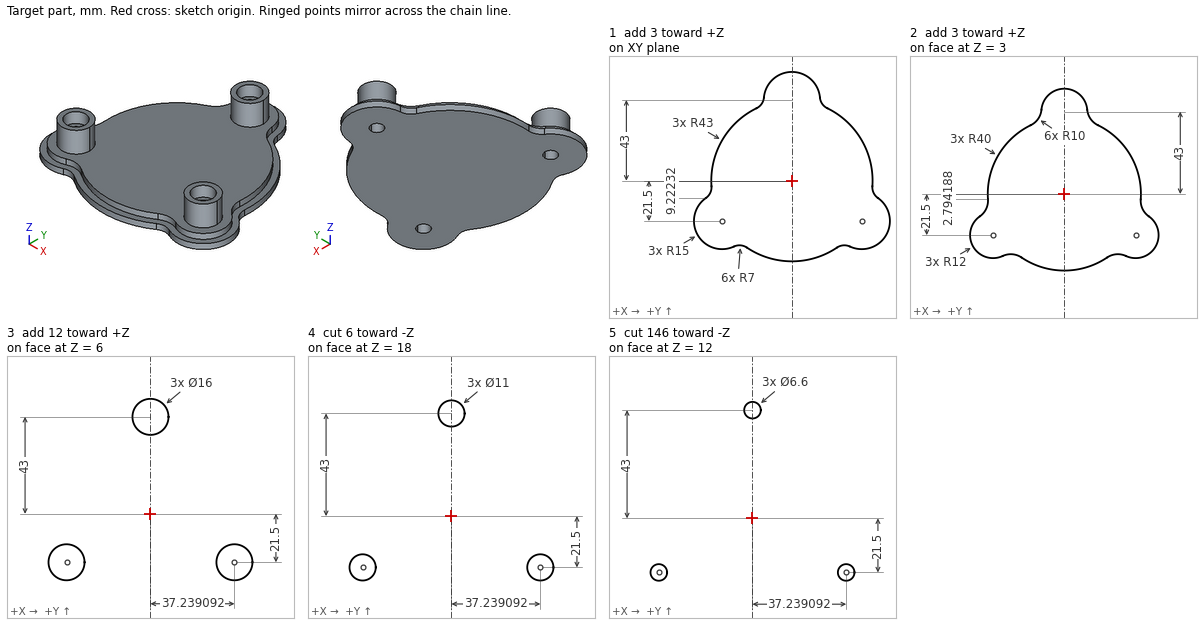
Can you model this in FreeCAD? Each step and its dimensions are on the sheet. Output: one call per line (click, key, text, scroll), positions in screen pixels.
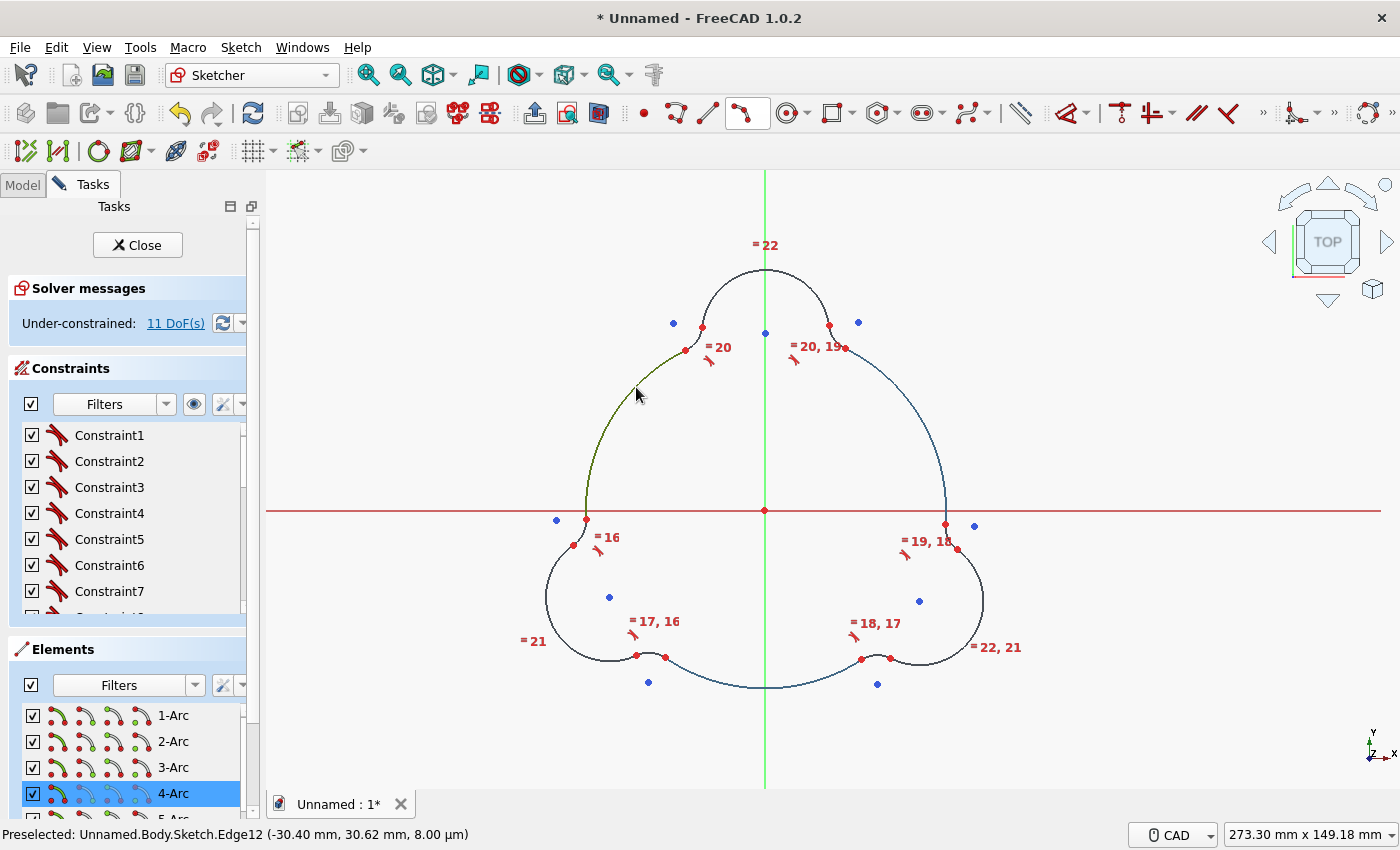
key(e)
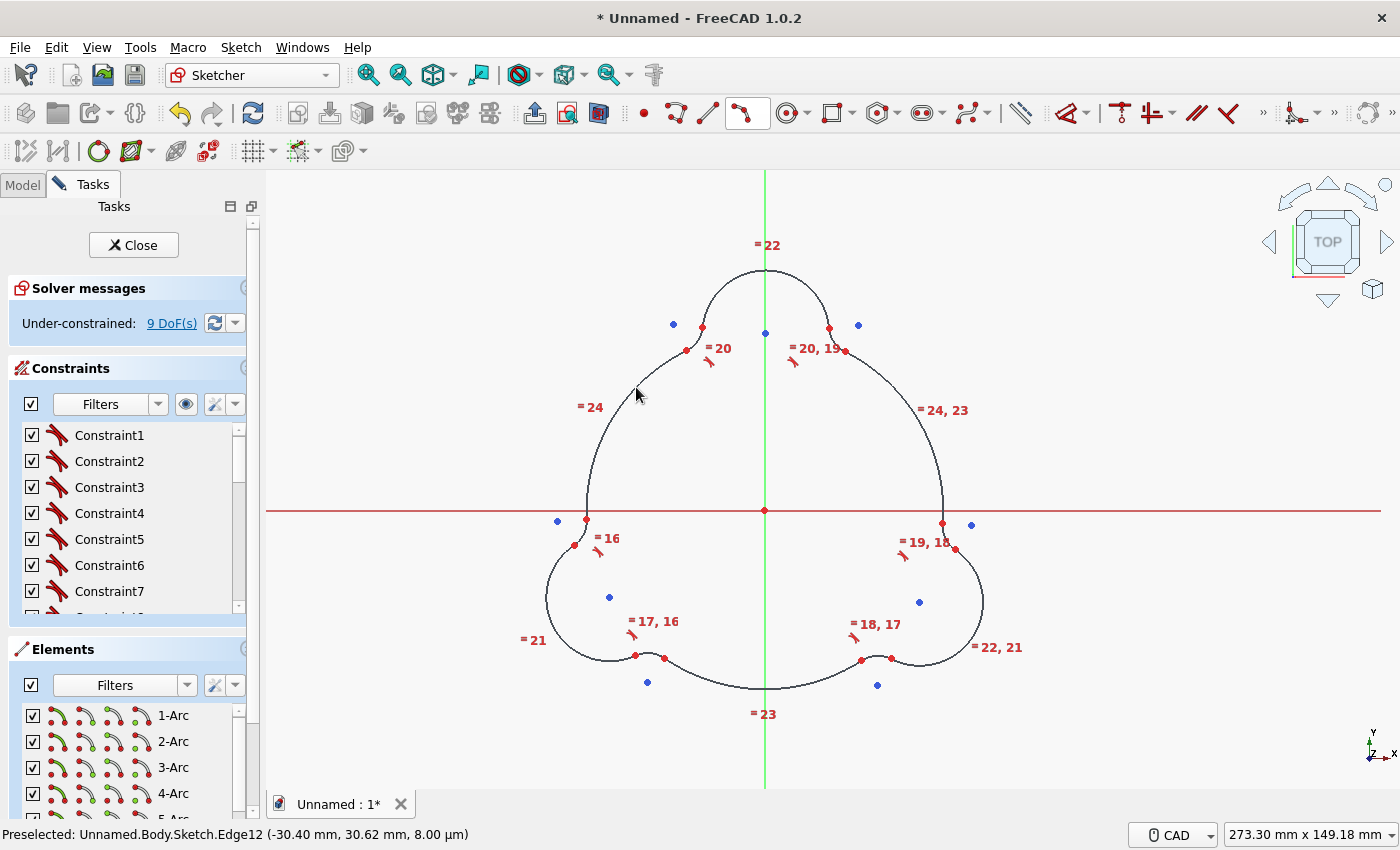
click(766, 334)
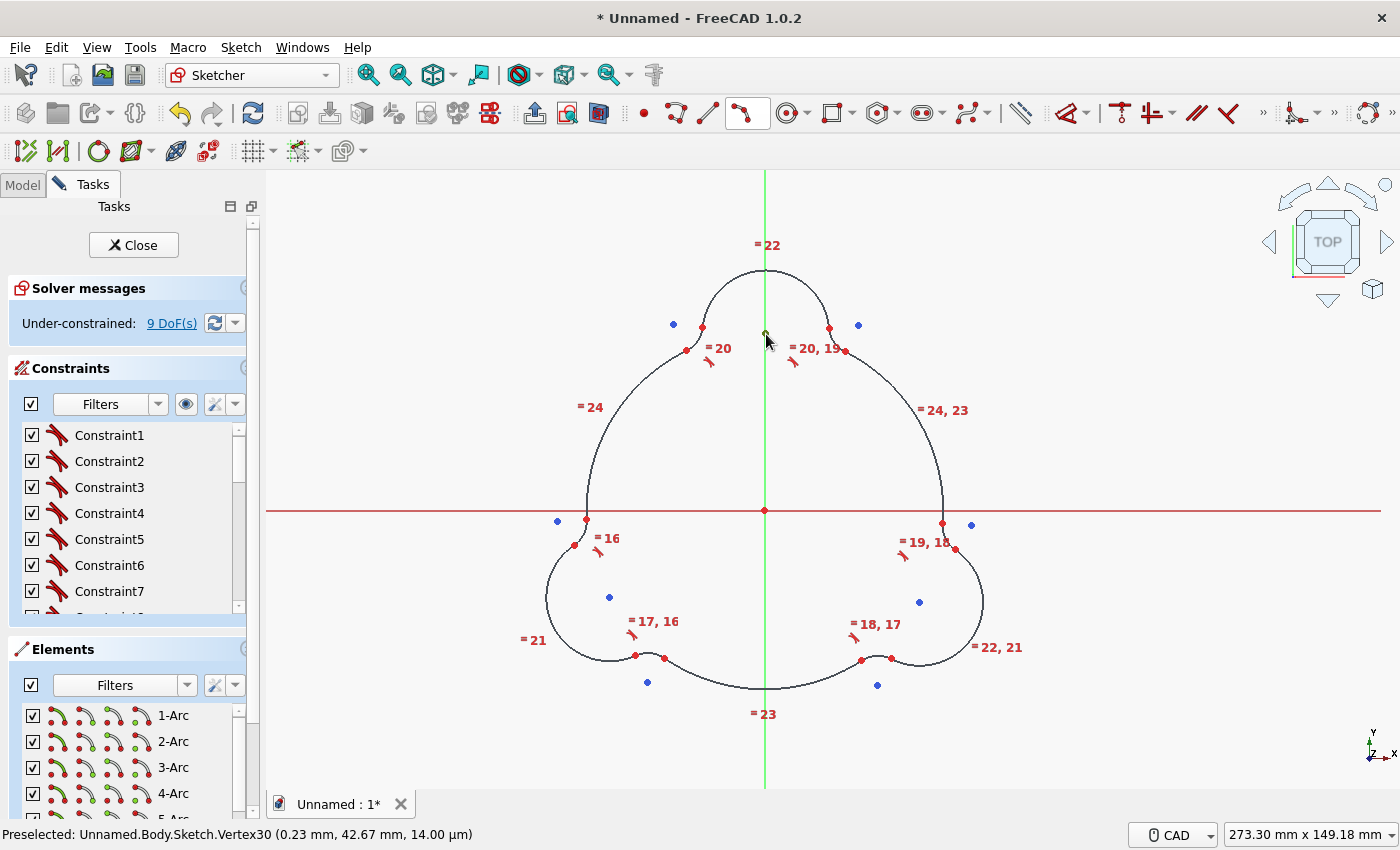
click(765, 721)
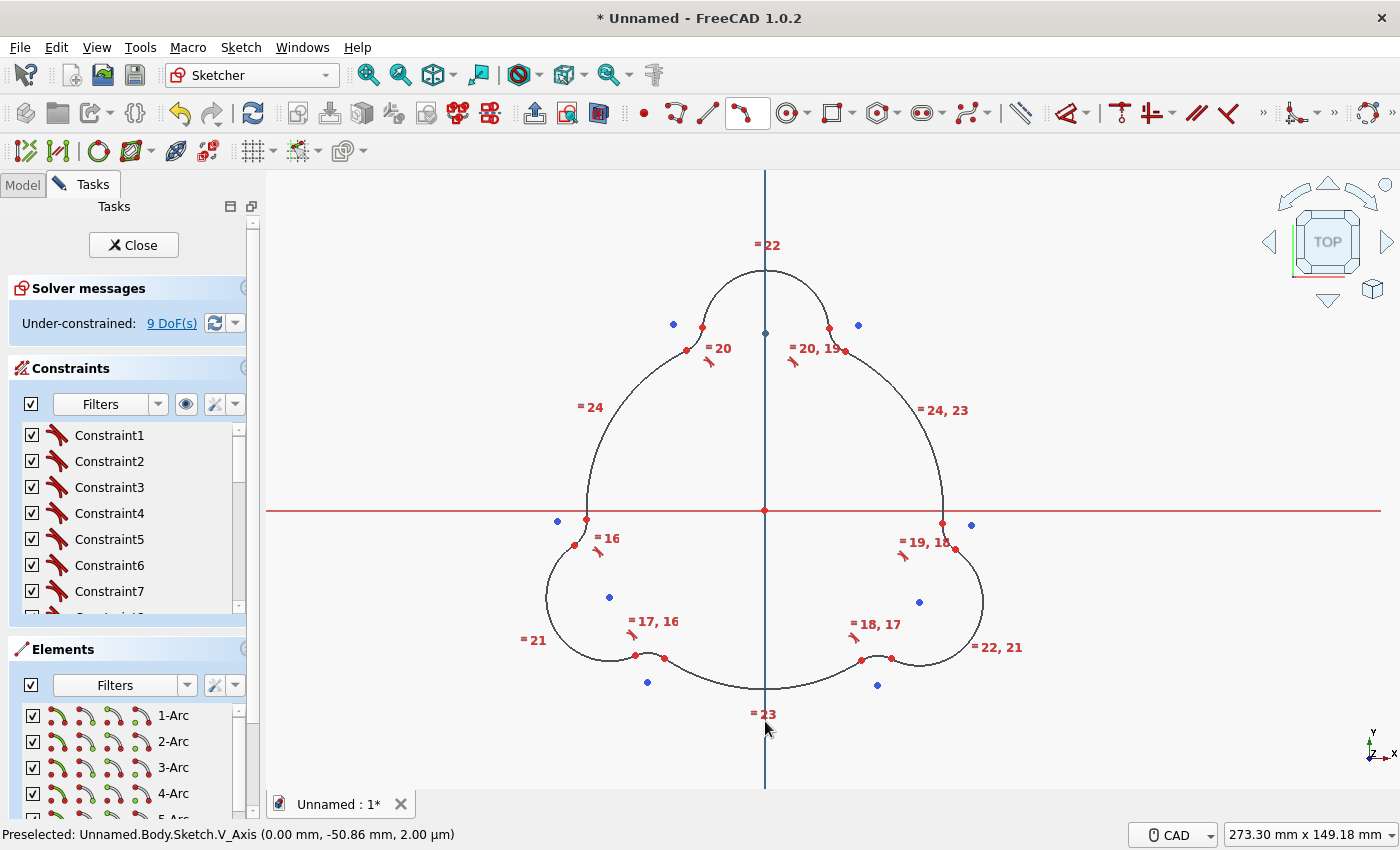
click(1120, 114)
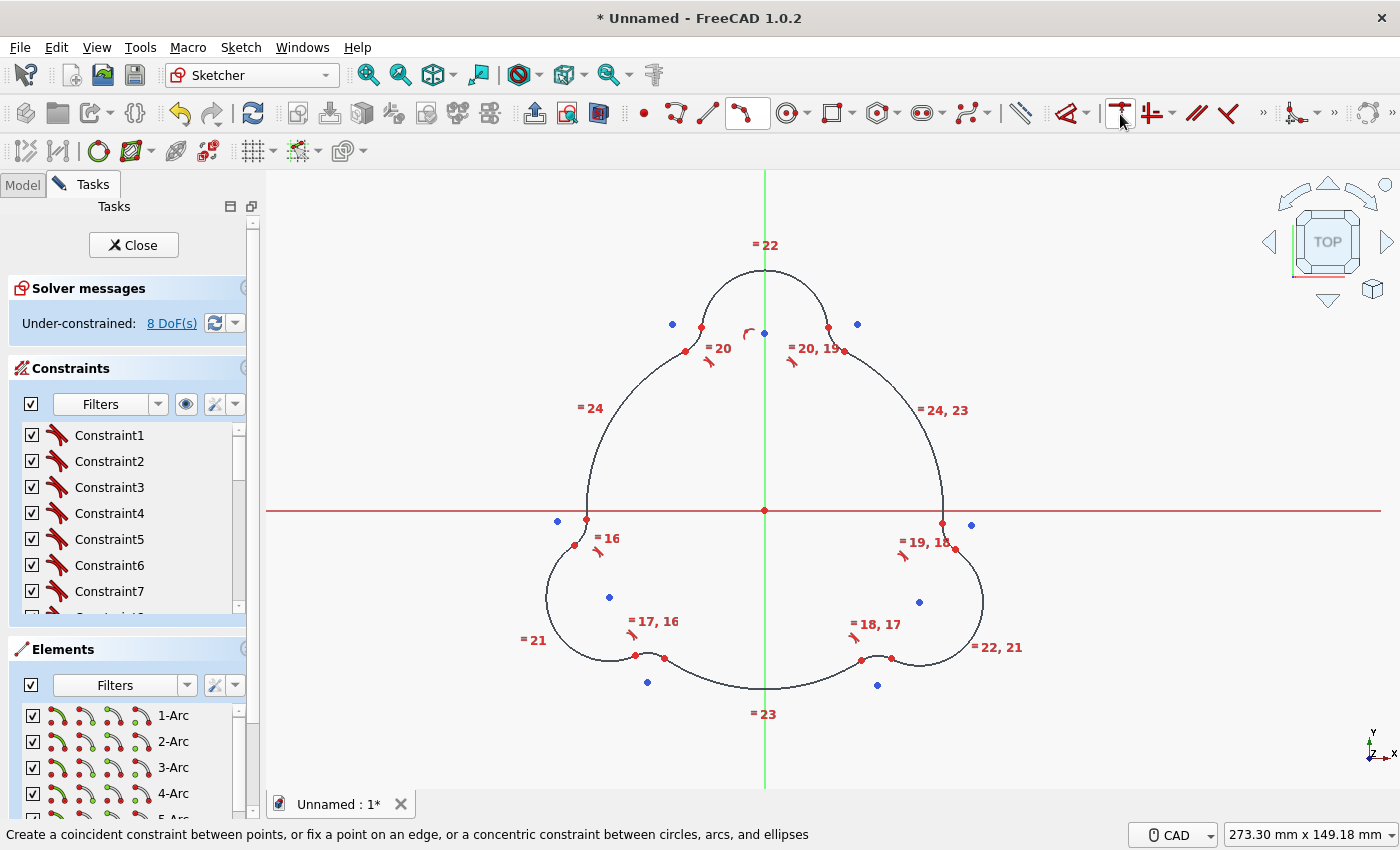
click(610, 598)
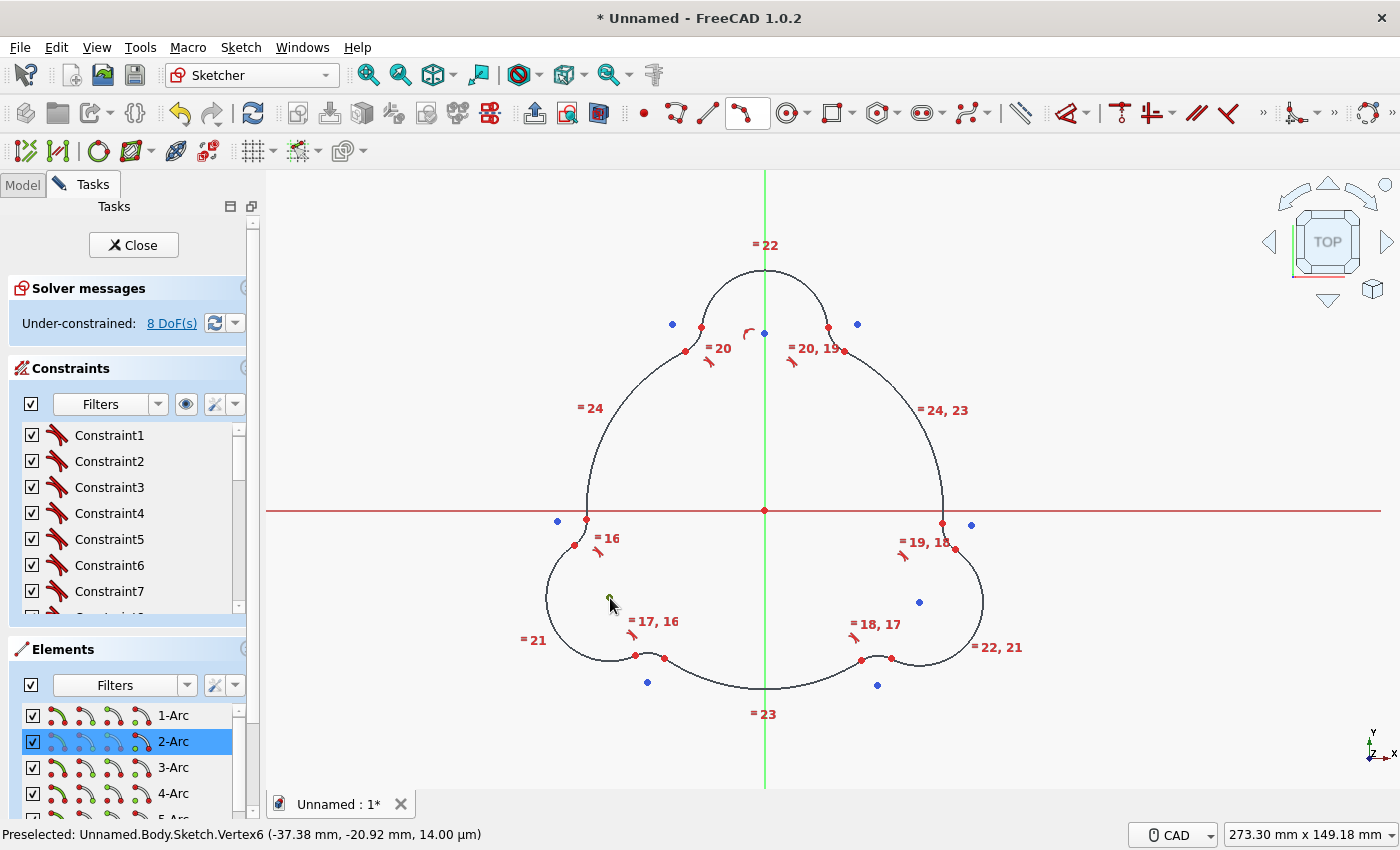
click(920, 602)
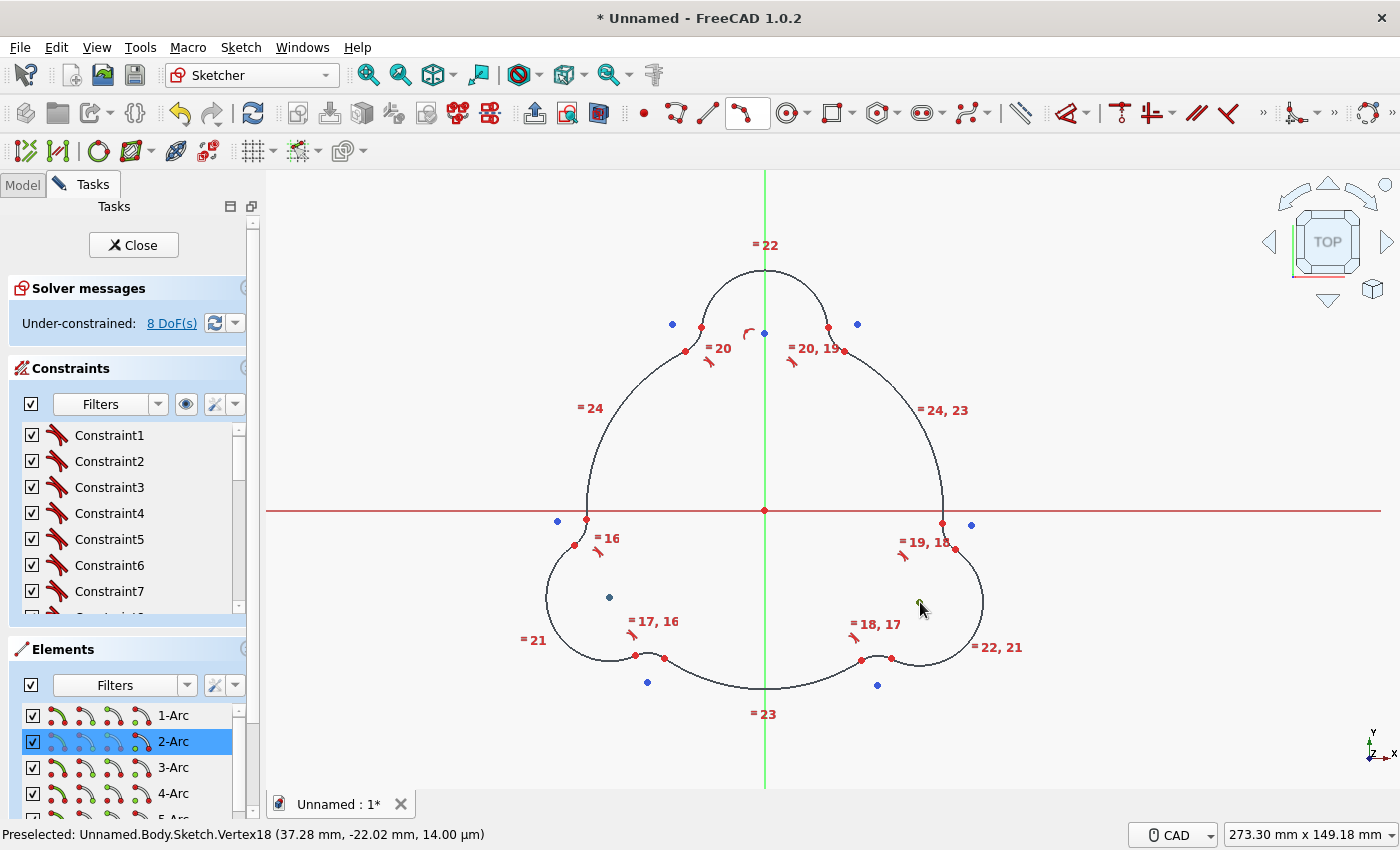
click(765, 721)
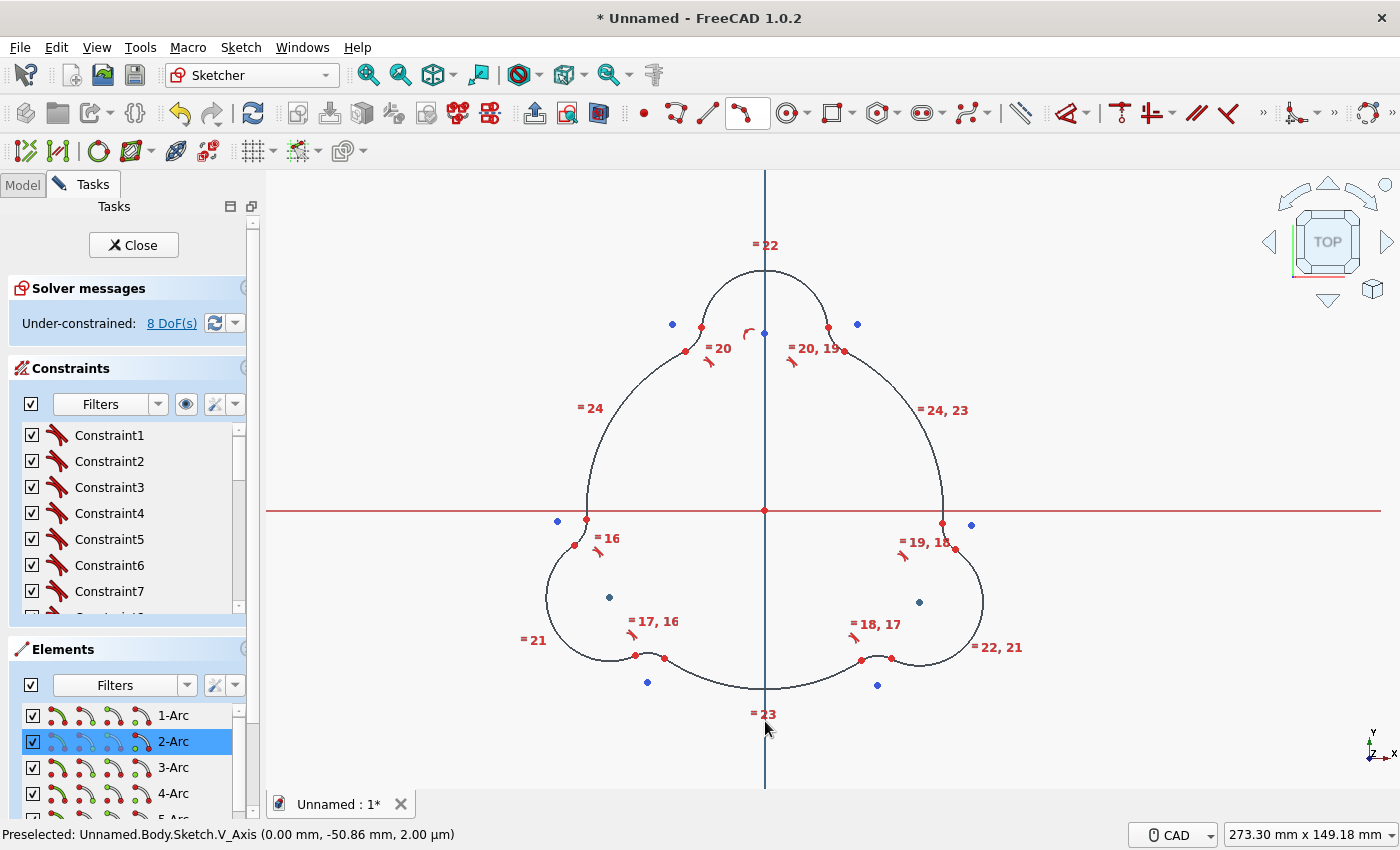
key(s)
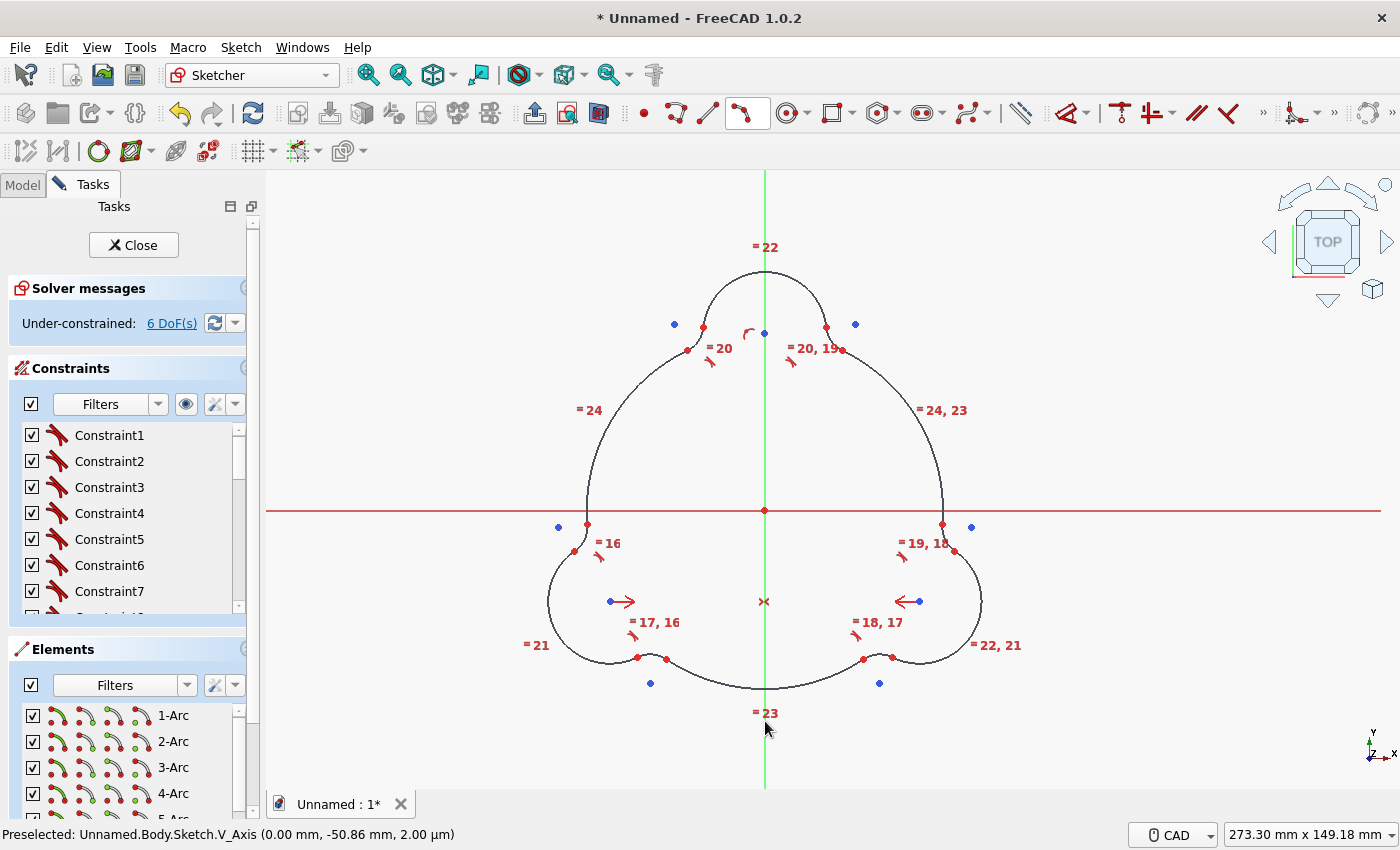
scroll(581, 545, up, 3)